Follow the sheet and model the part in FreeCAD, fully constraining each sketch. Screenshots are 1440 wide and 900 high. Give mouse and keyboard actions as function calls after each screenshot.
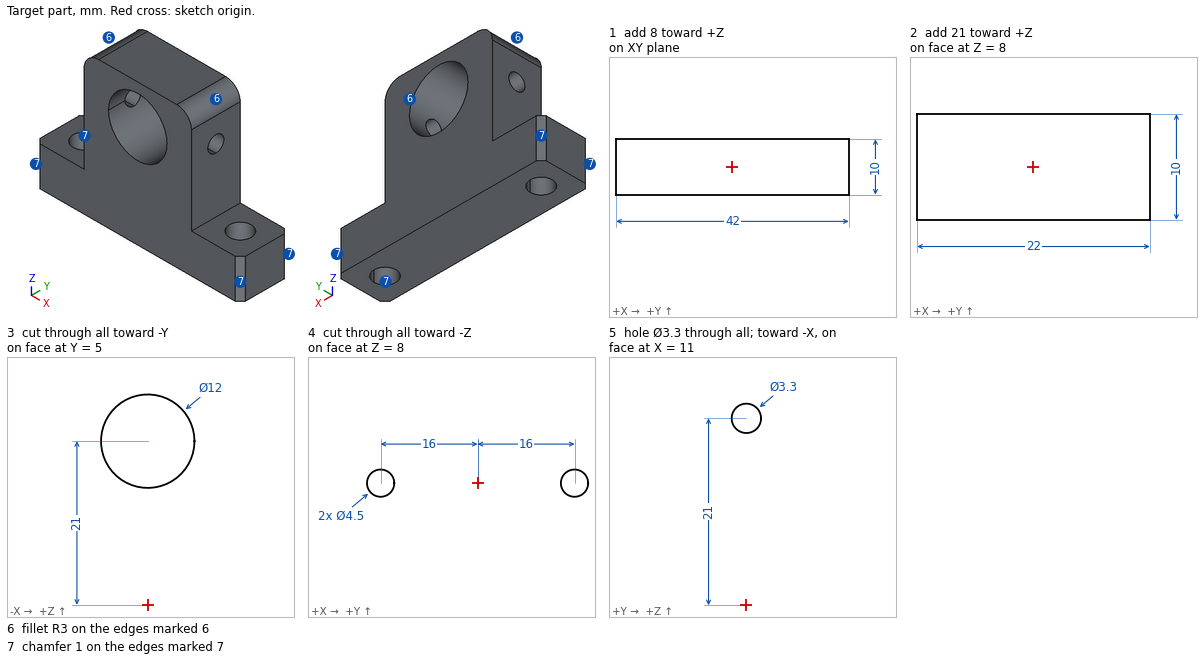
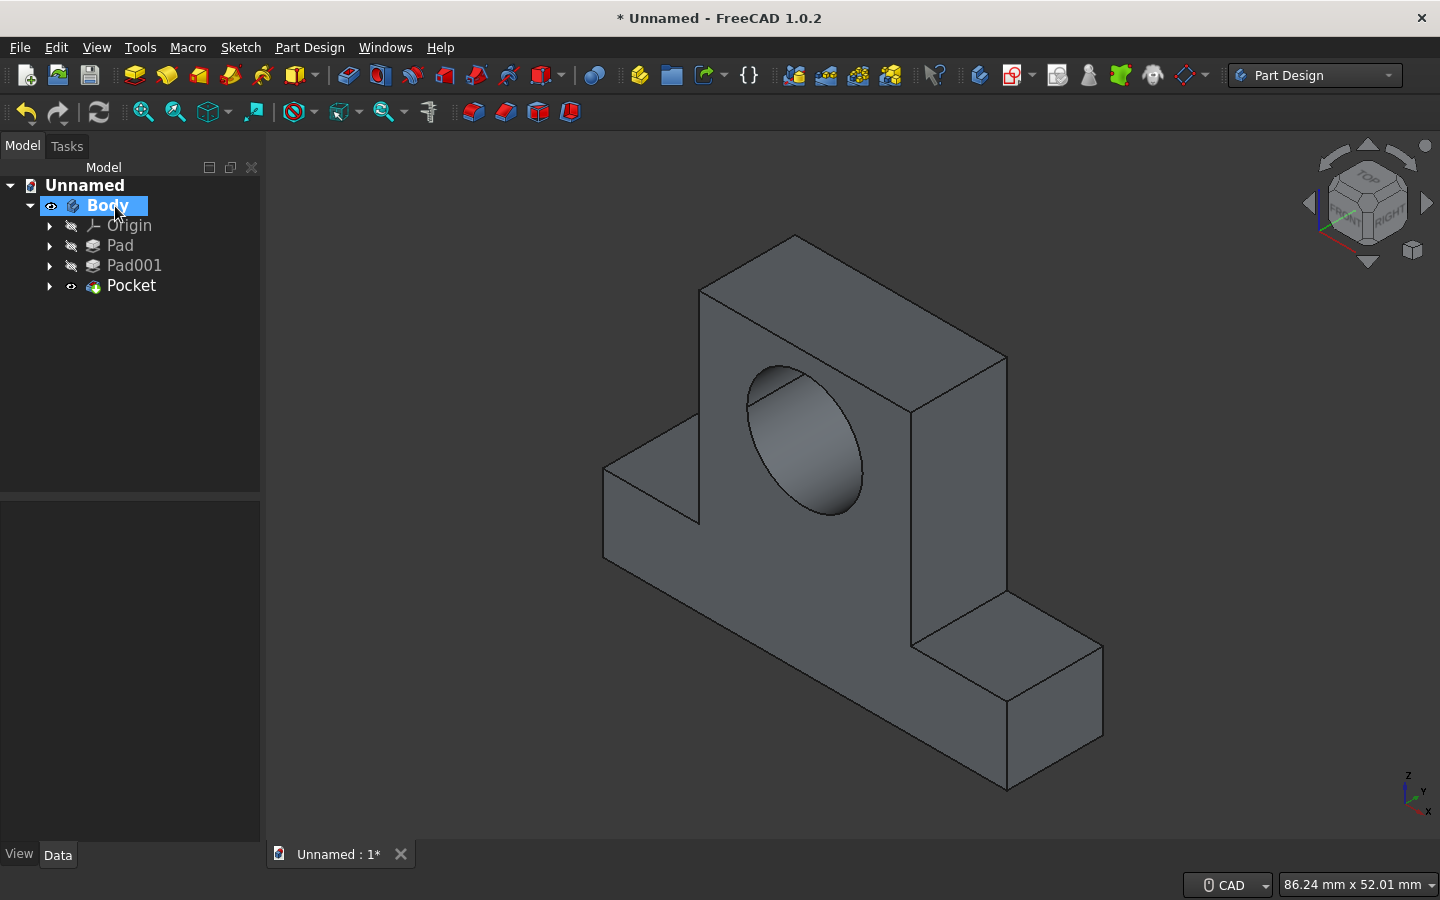
click(685, 459)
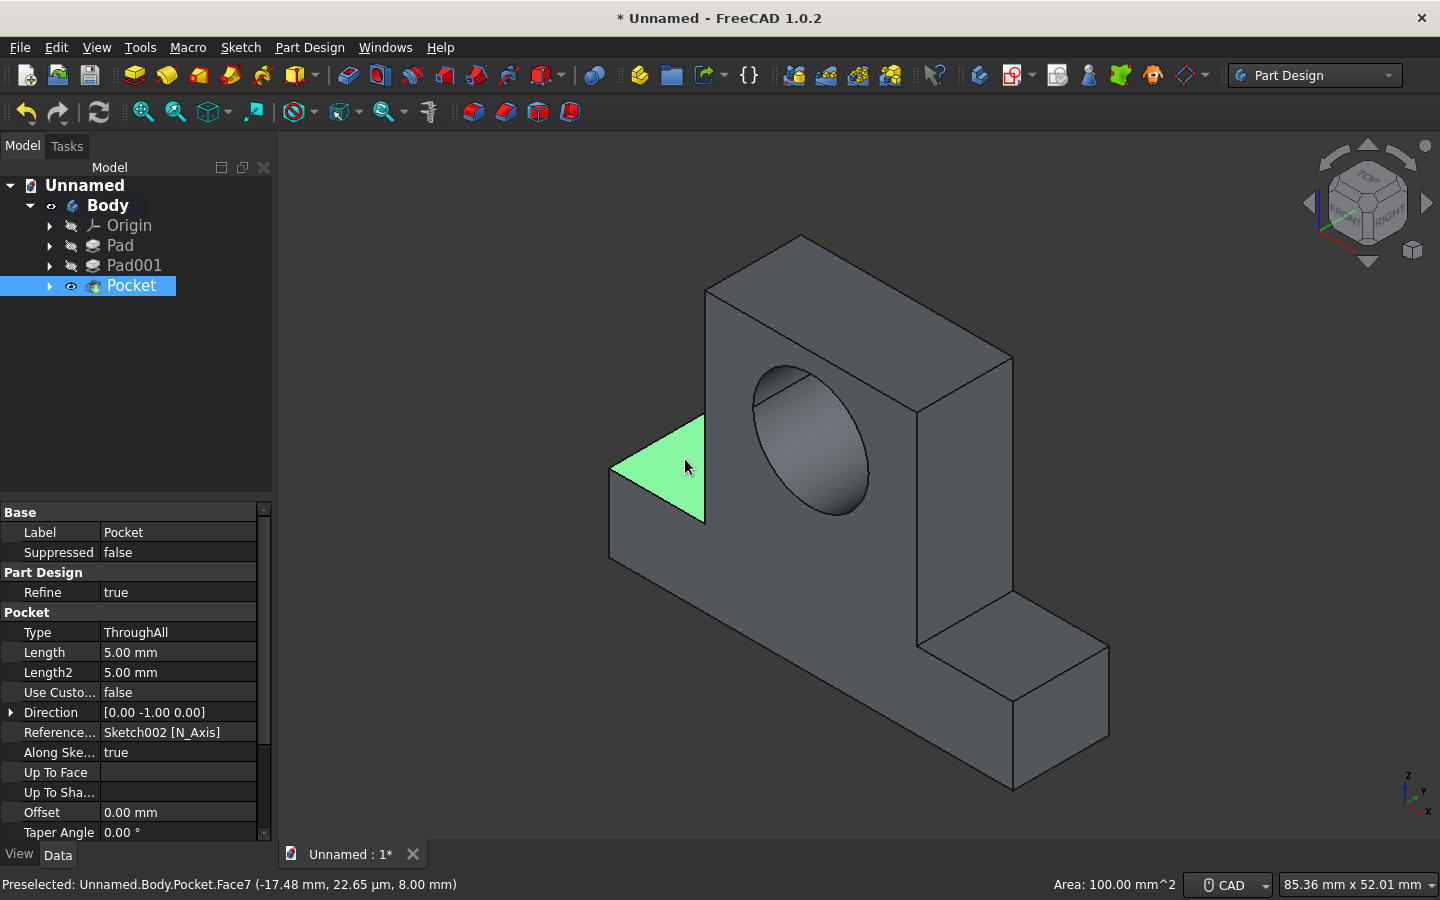
click(1012, 76)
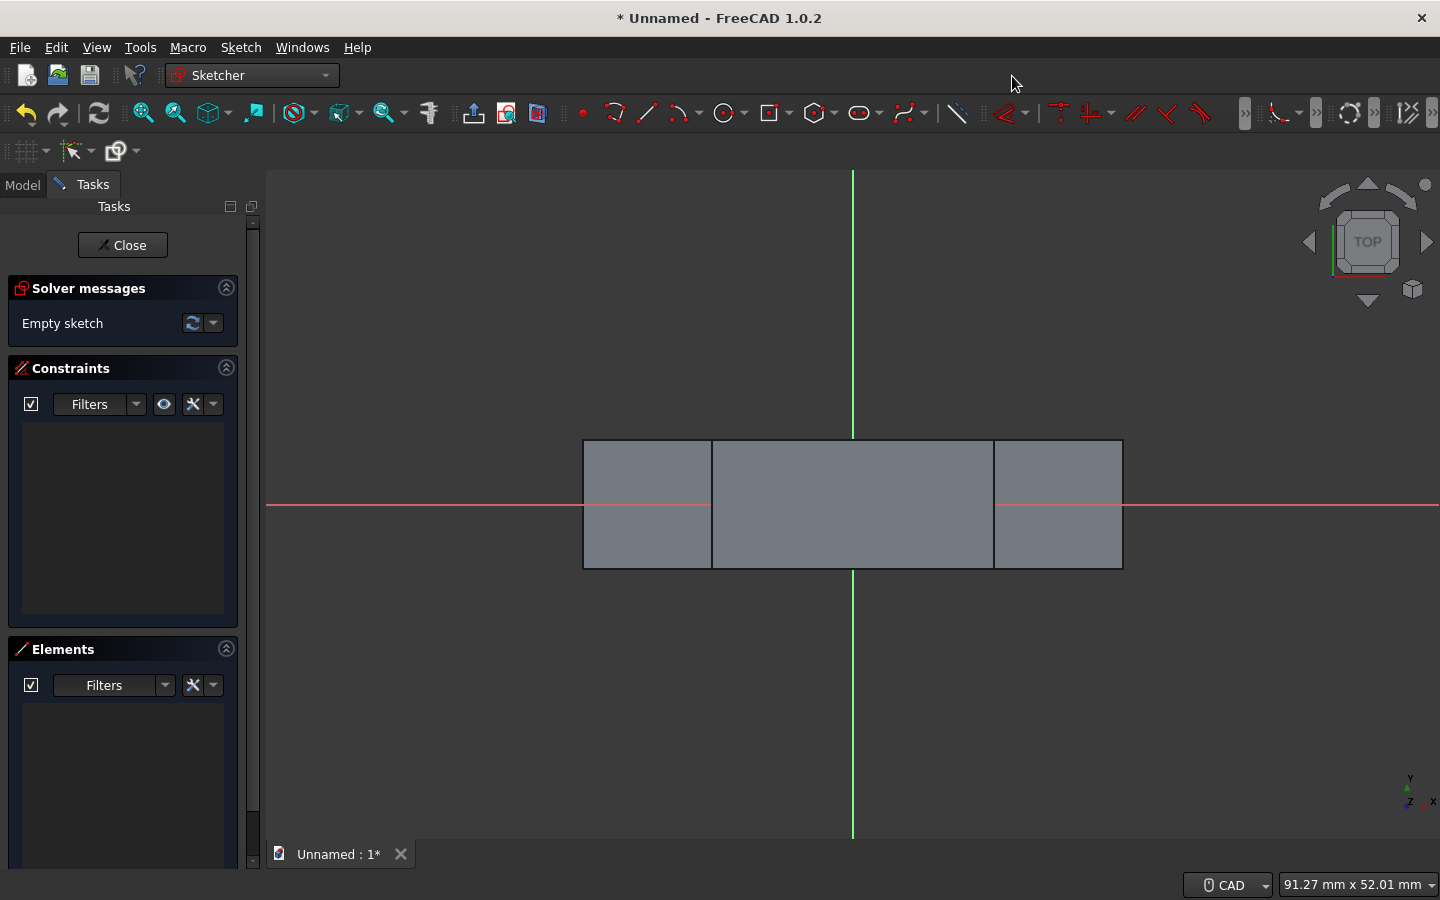
key(q)
key(s)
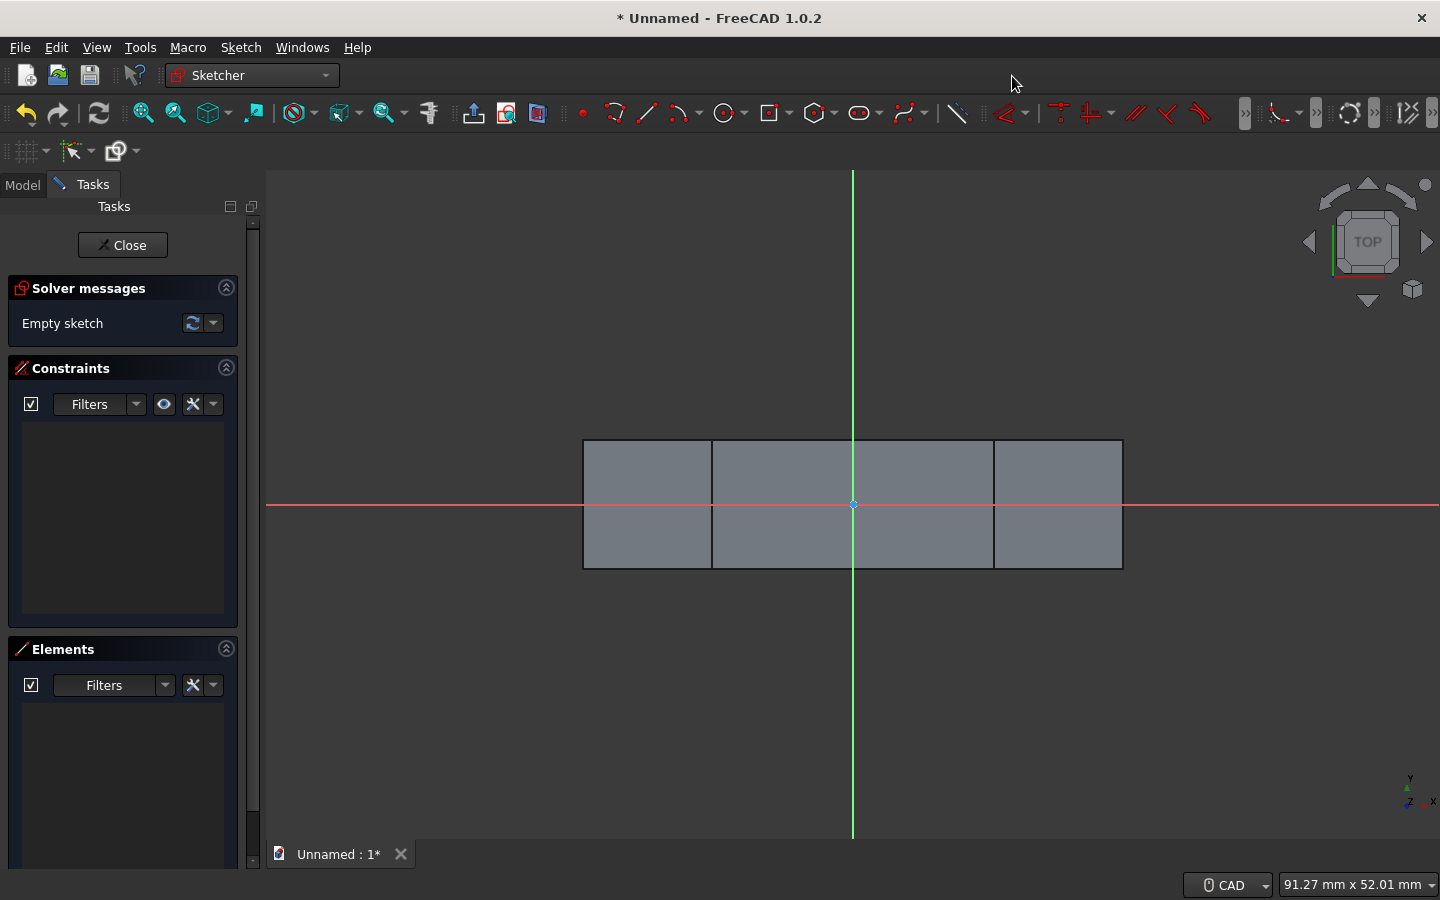
scroll(992, 504, up, 2)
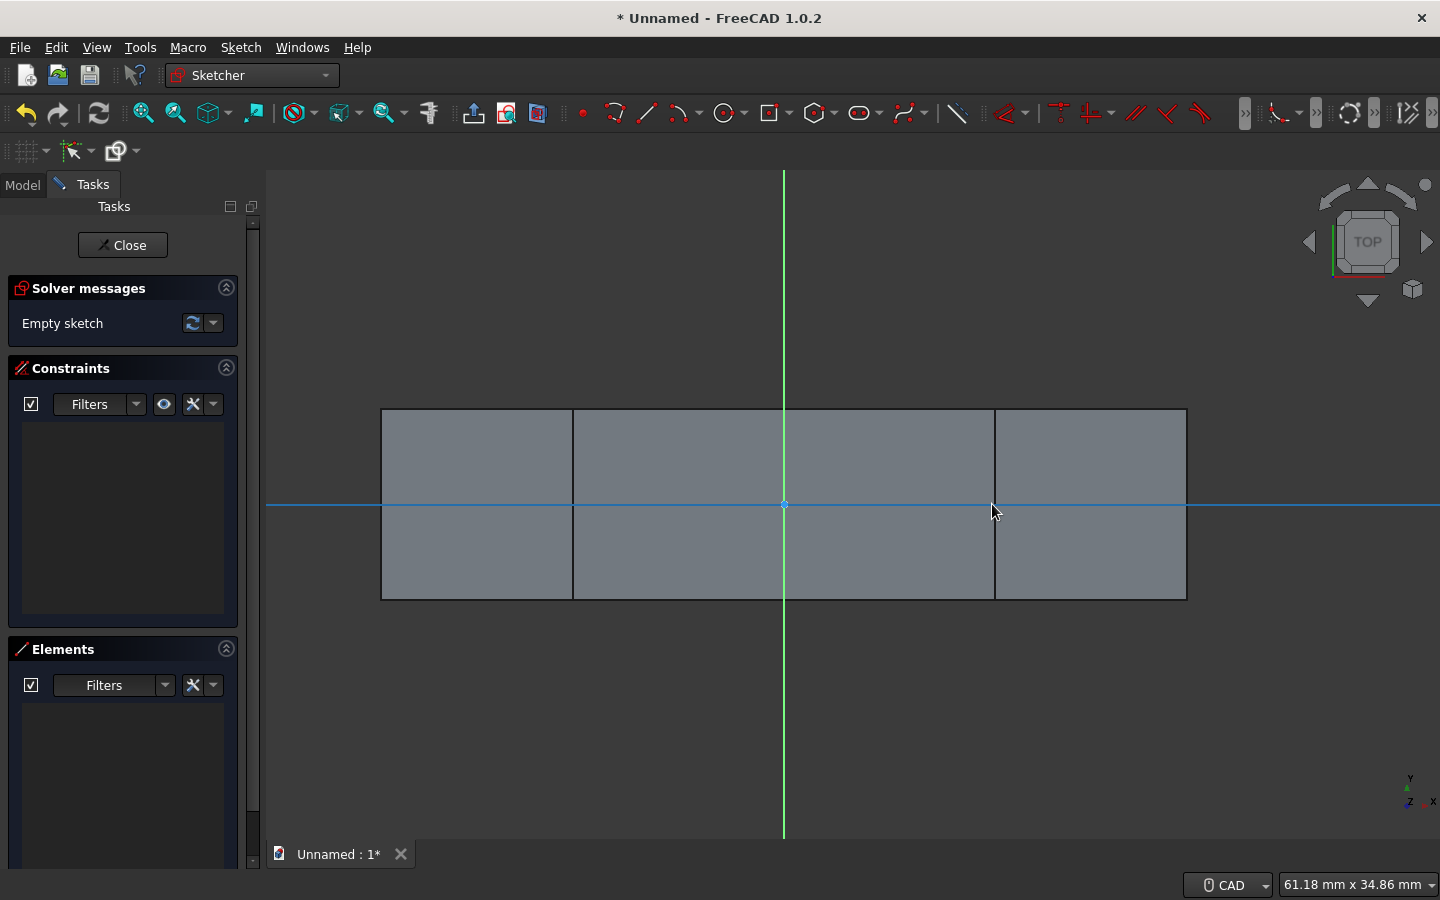
click(724, 114)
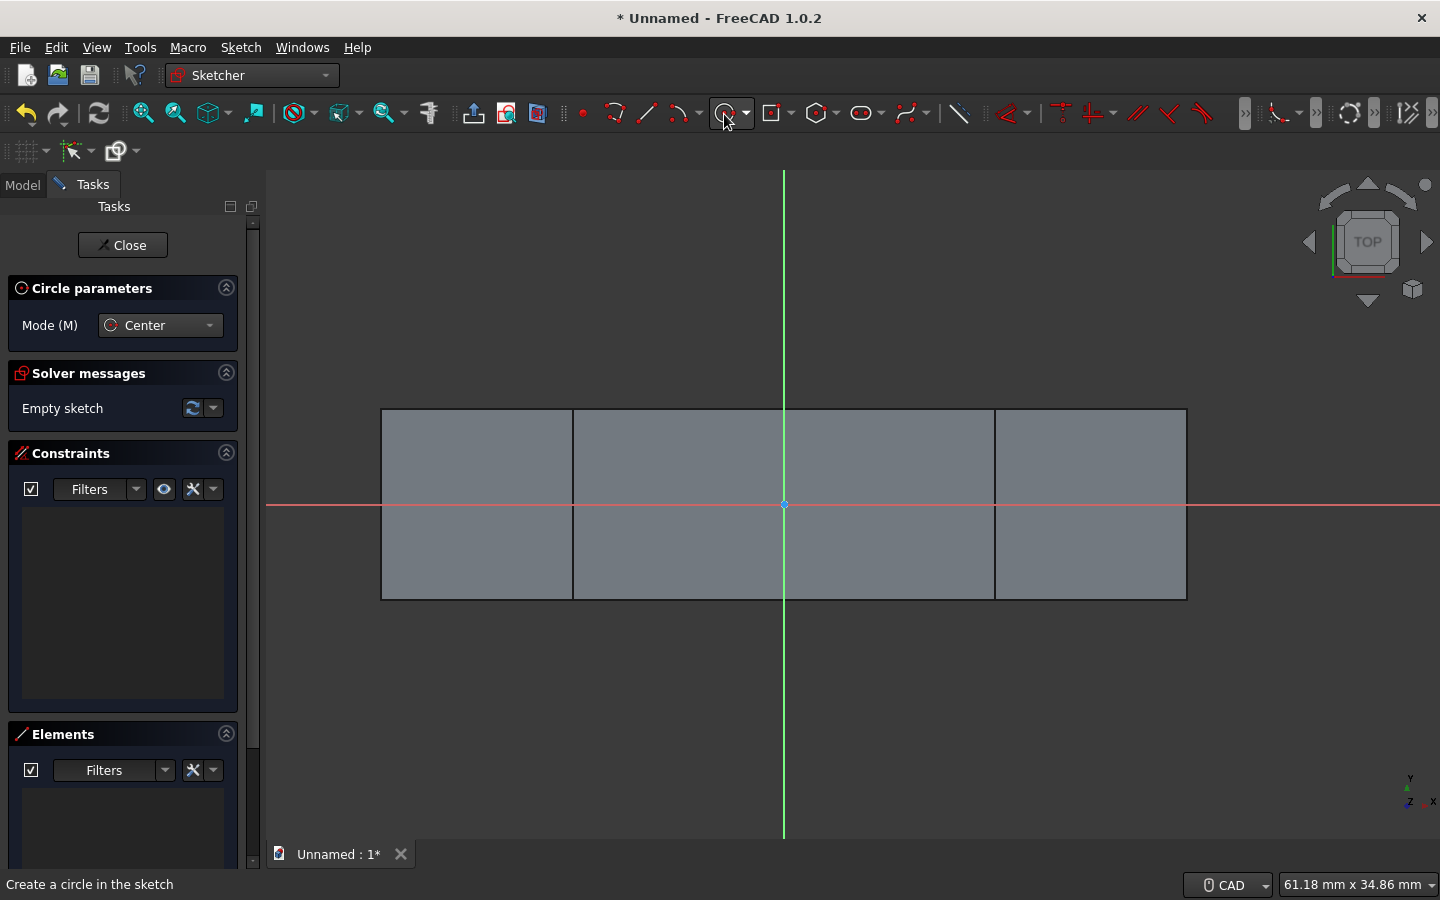
click(477, 504)
click(508, 474)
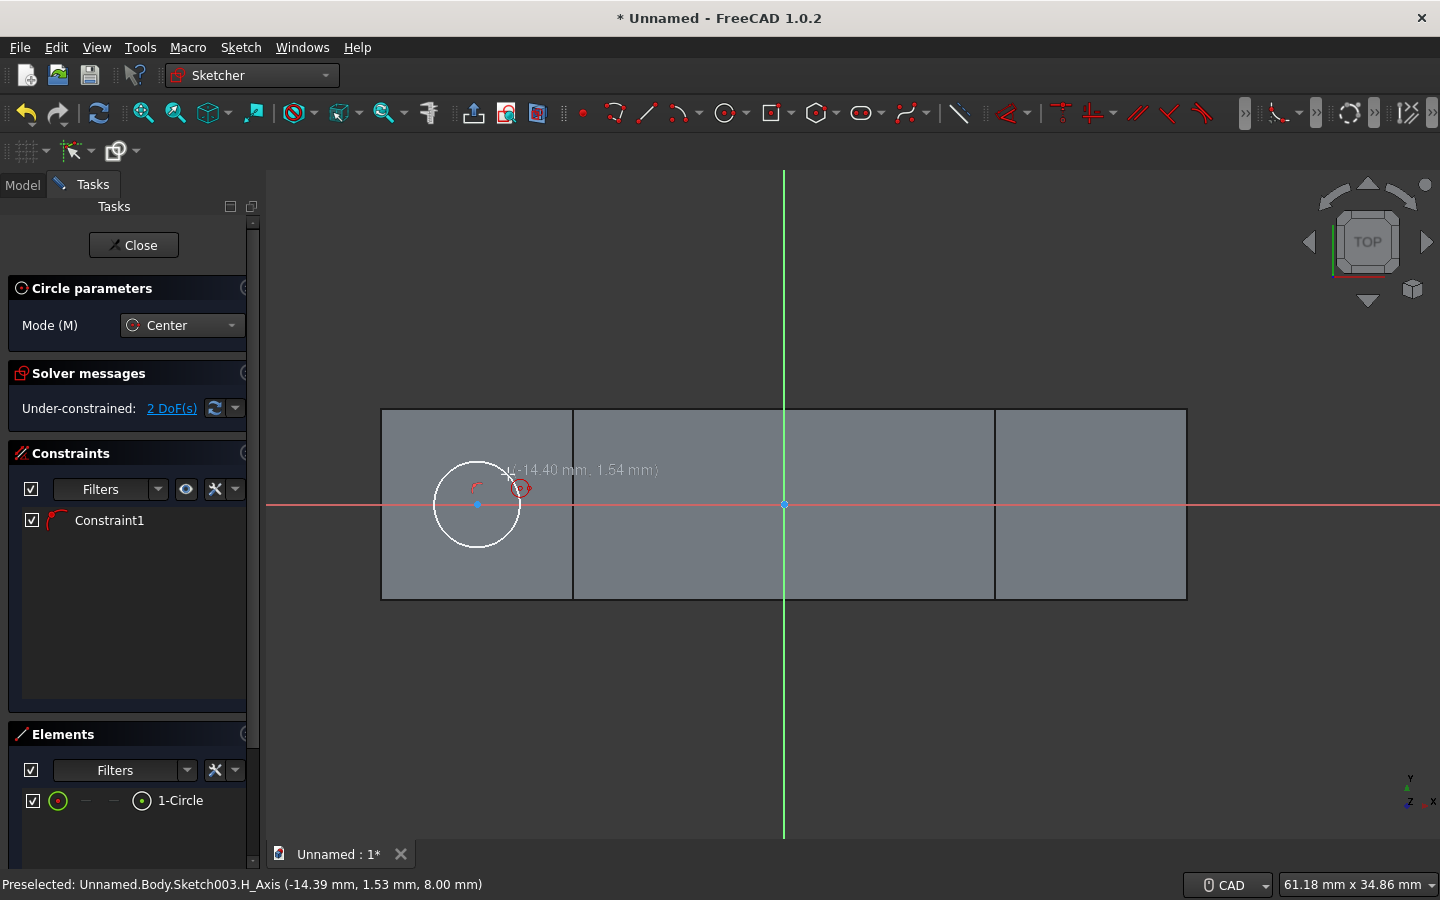
click(1091, 504)
click(1122, 474)
key(Escape)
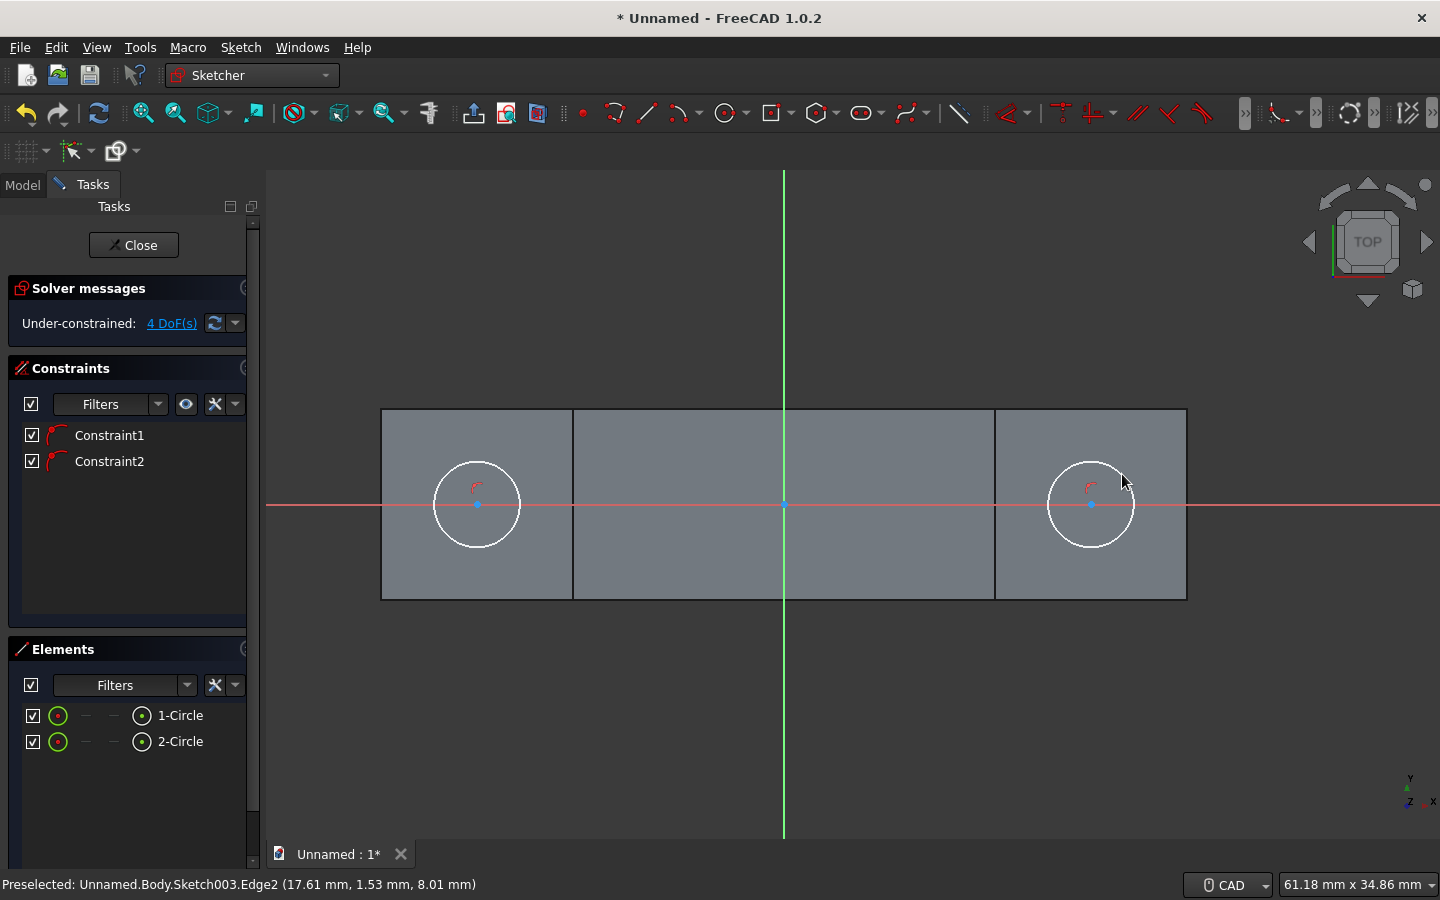
click(507, 474)